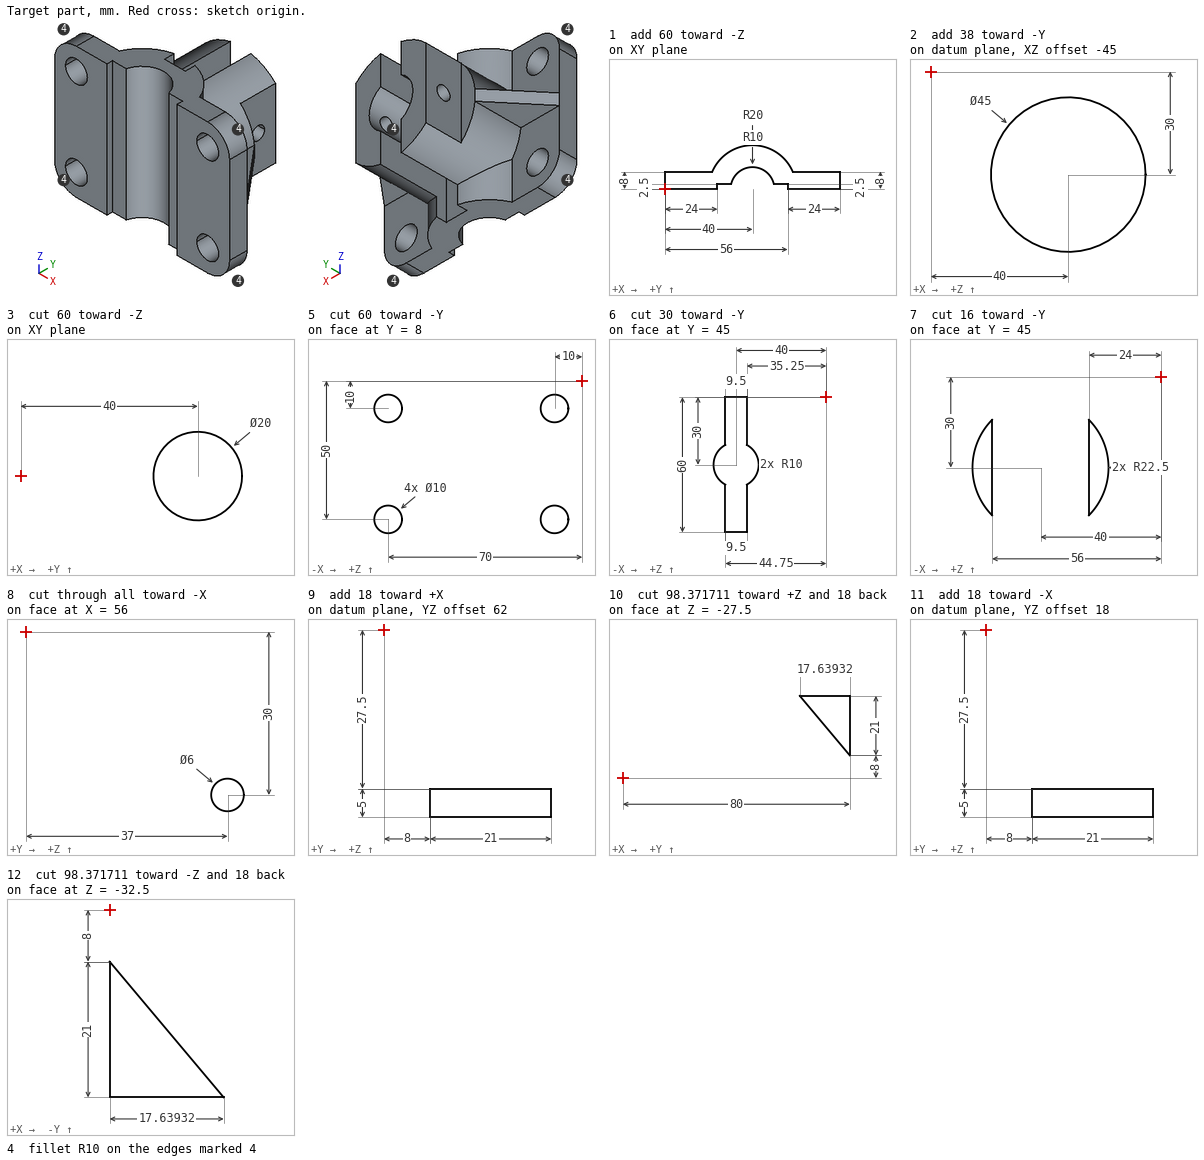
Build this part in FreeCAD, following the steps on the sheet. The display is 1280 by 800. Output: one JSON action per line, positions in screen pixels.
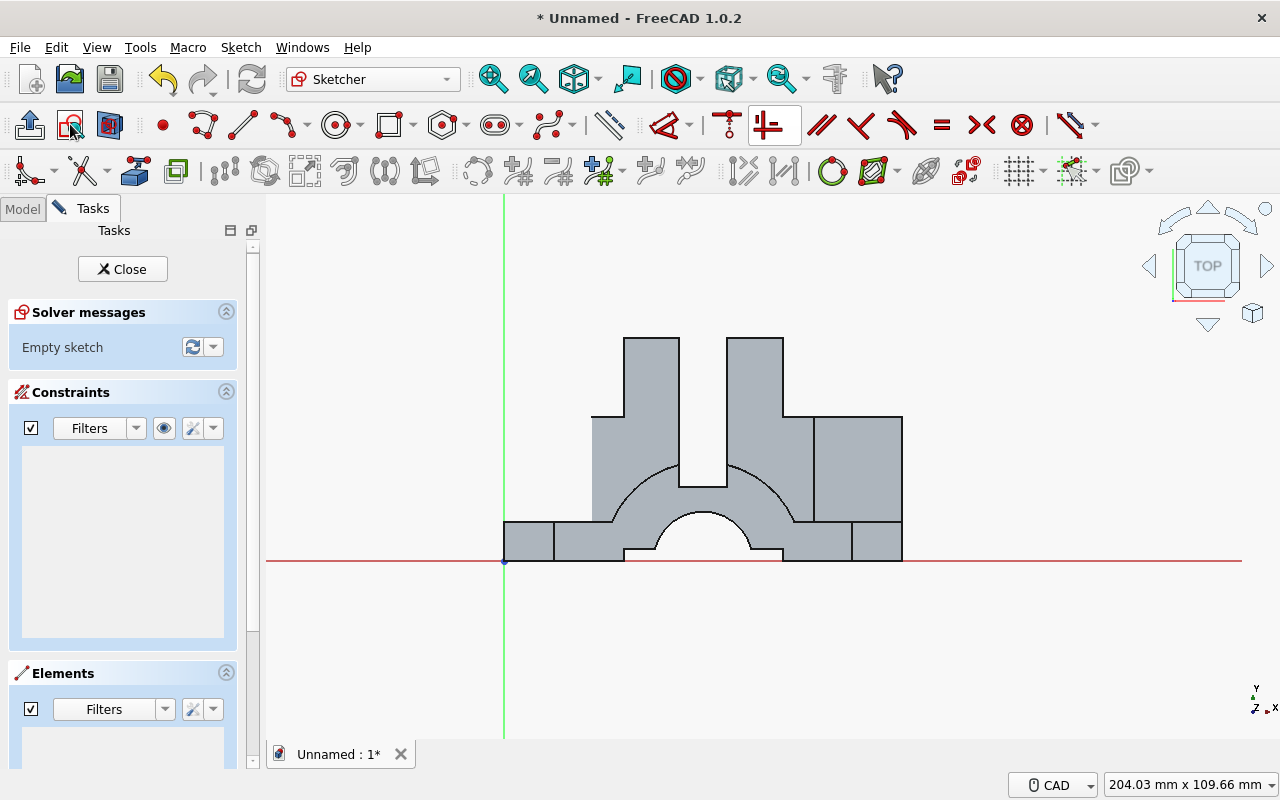
{"action": "left_click", "coordinate": [110, 126]}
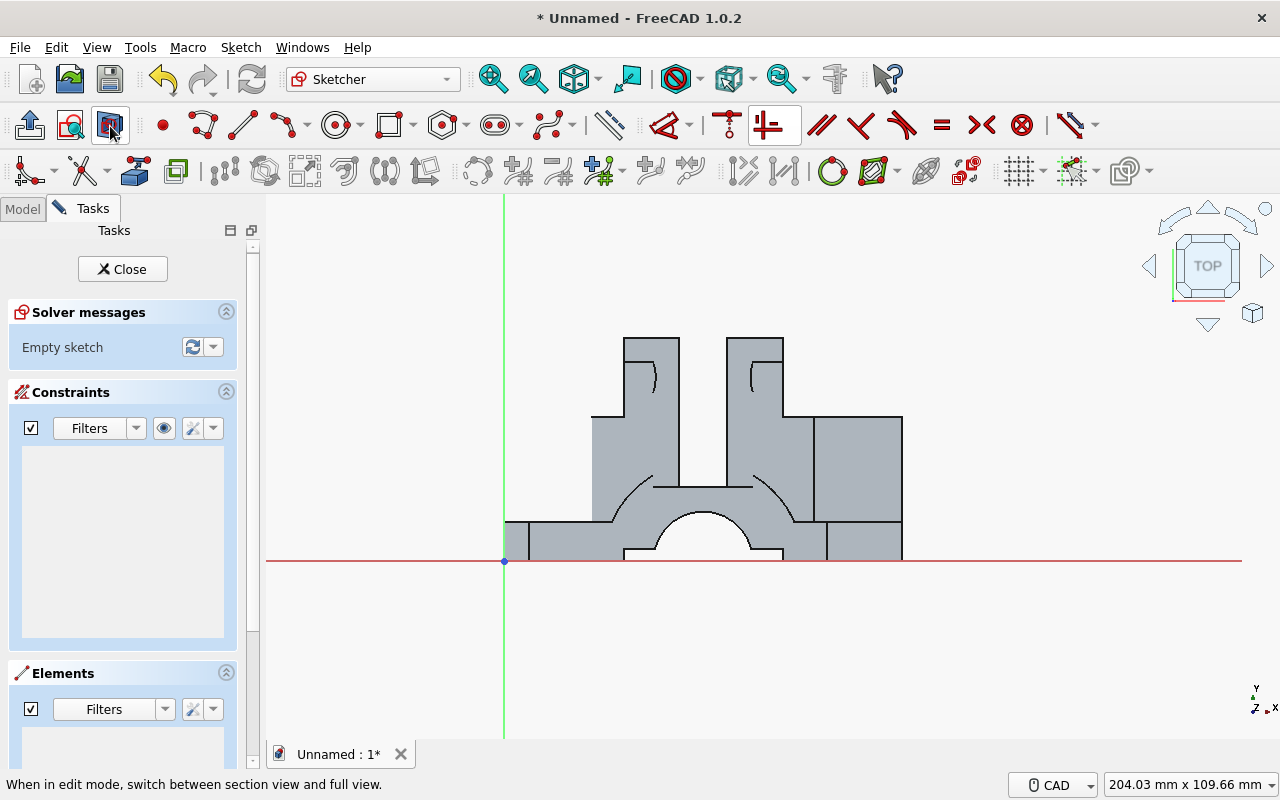
{"action": "scroll", "coordinate": [924, 471], "scroll_direction": "up", "scroll_amount": 6}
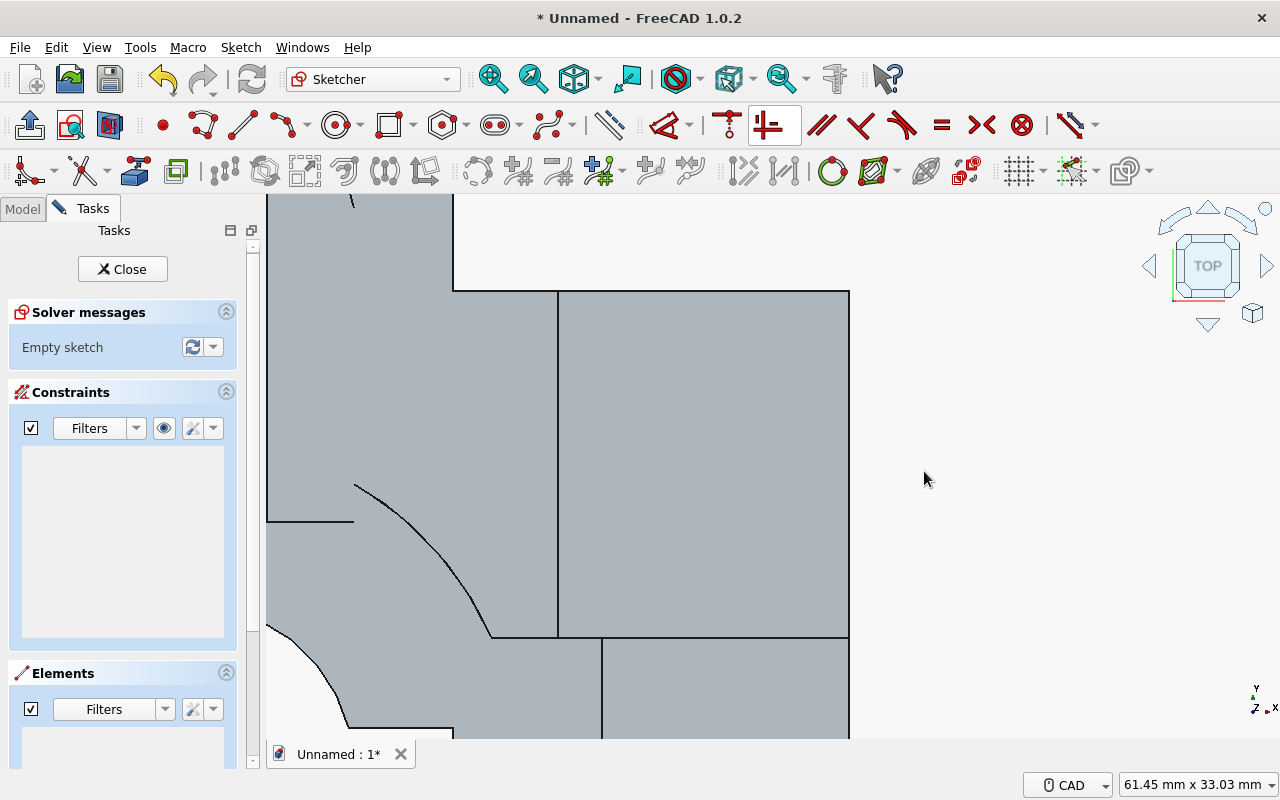
{"action": "left_click", "coordinate": [204, 126]}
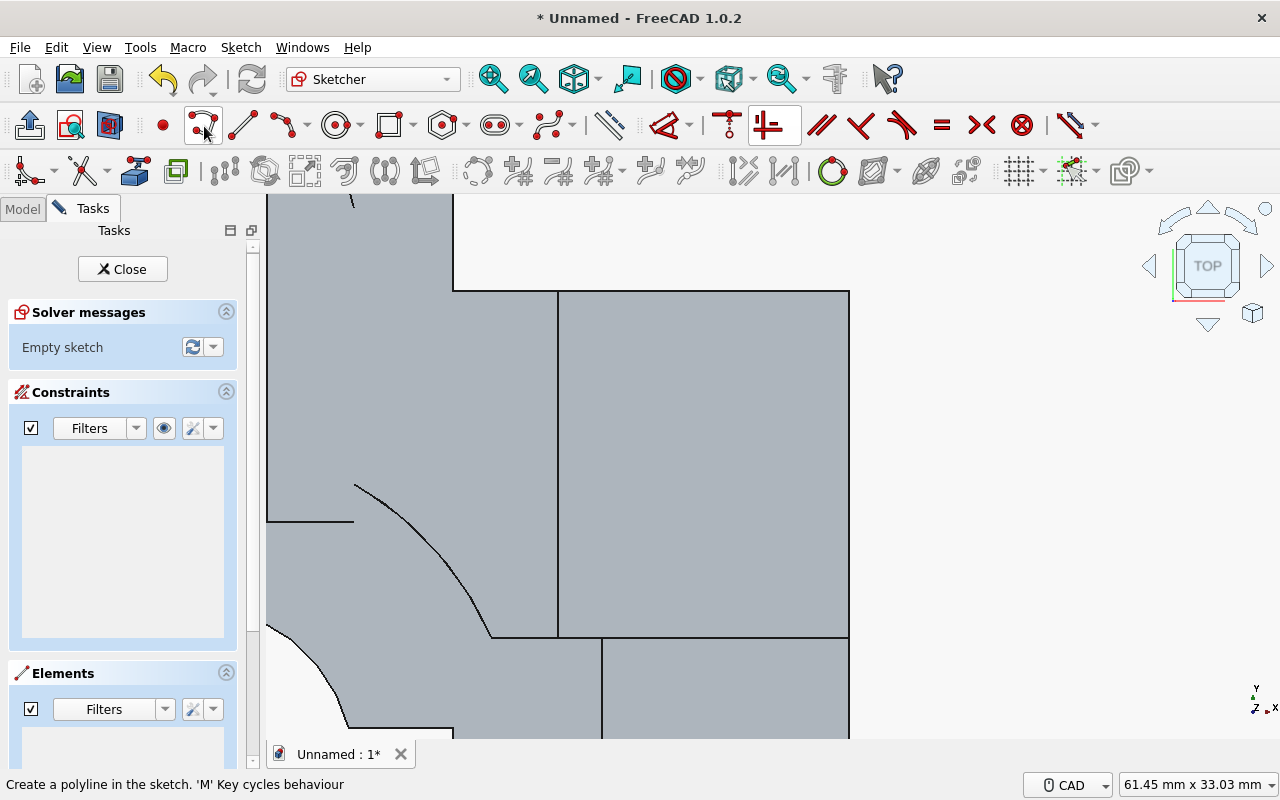
{"action": "left_click", "coordinate": [558, 291]}
{"action": "left_click", "coordinate": [849, 638]}
{"action": "left_click", "coordinate": [849, 291]}
{"action": "left_click", "coordinate": [558, 292]}
{"action": "key", "text": "Escape"}
{"action": "key", "text": "Escape"}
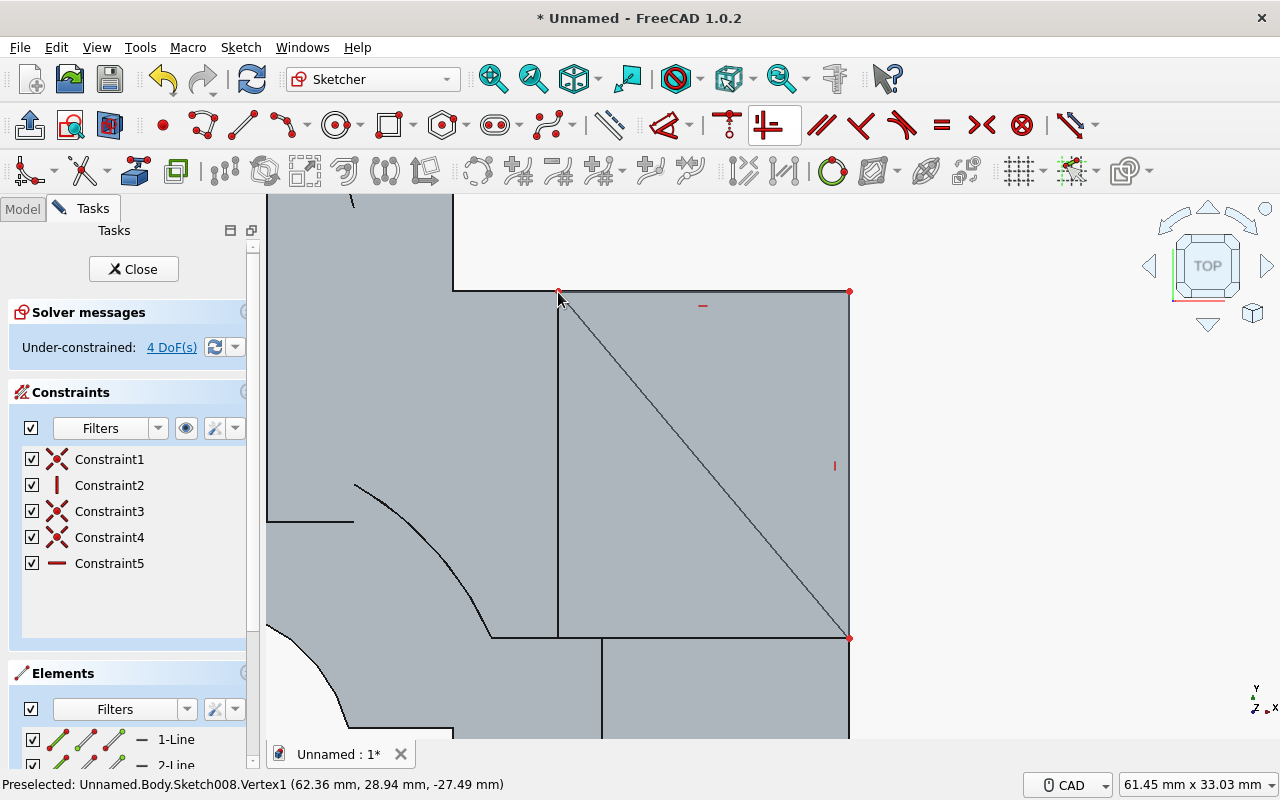
{"action": "left_click", "coordinate": [664, 126]}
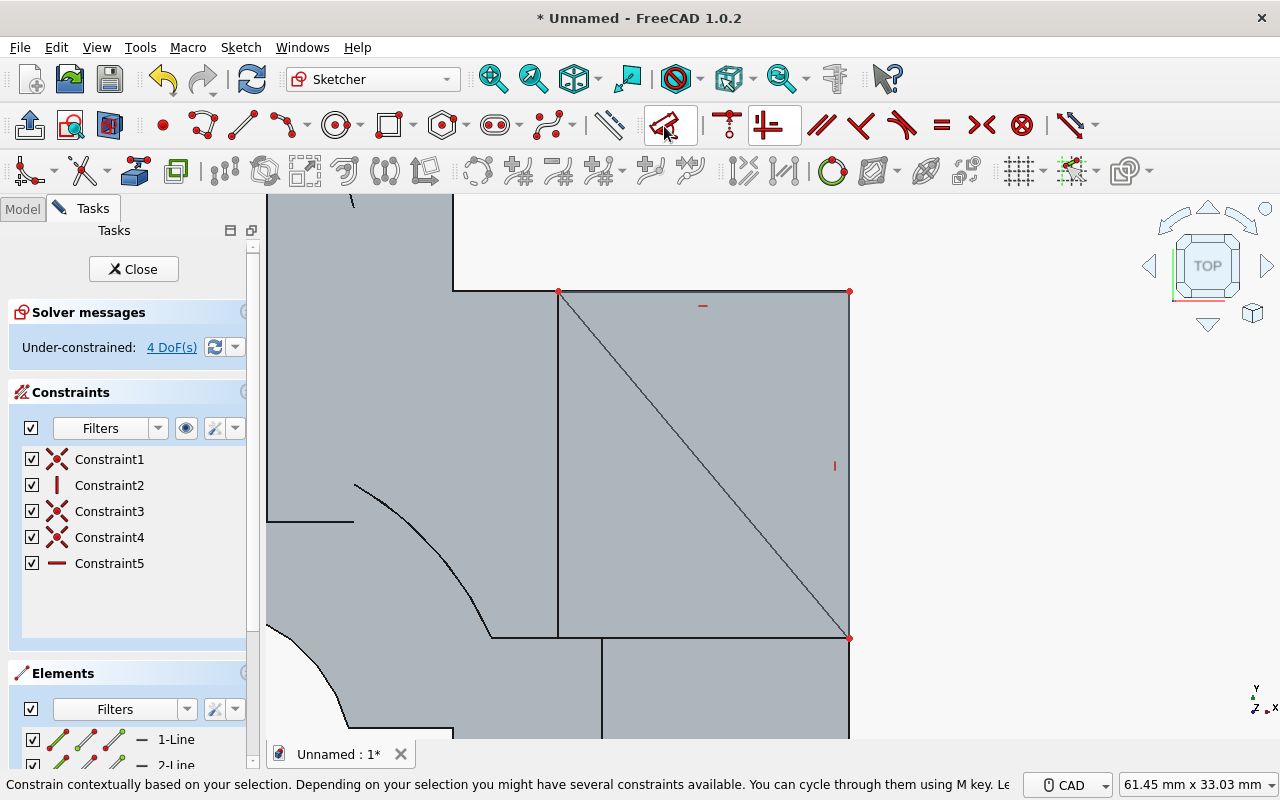
{"action": "left_click", "coordinate": [849, 535]}
{"action": "left_click", "coordinate": [883, 465]}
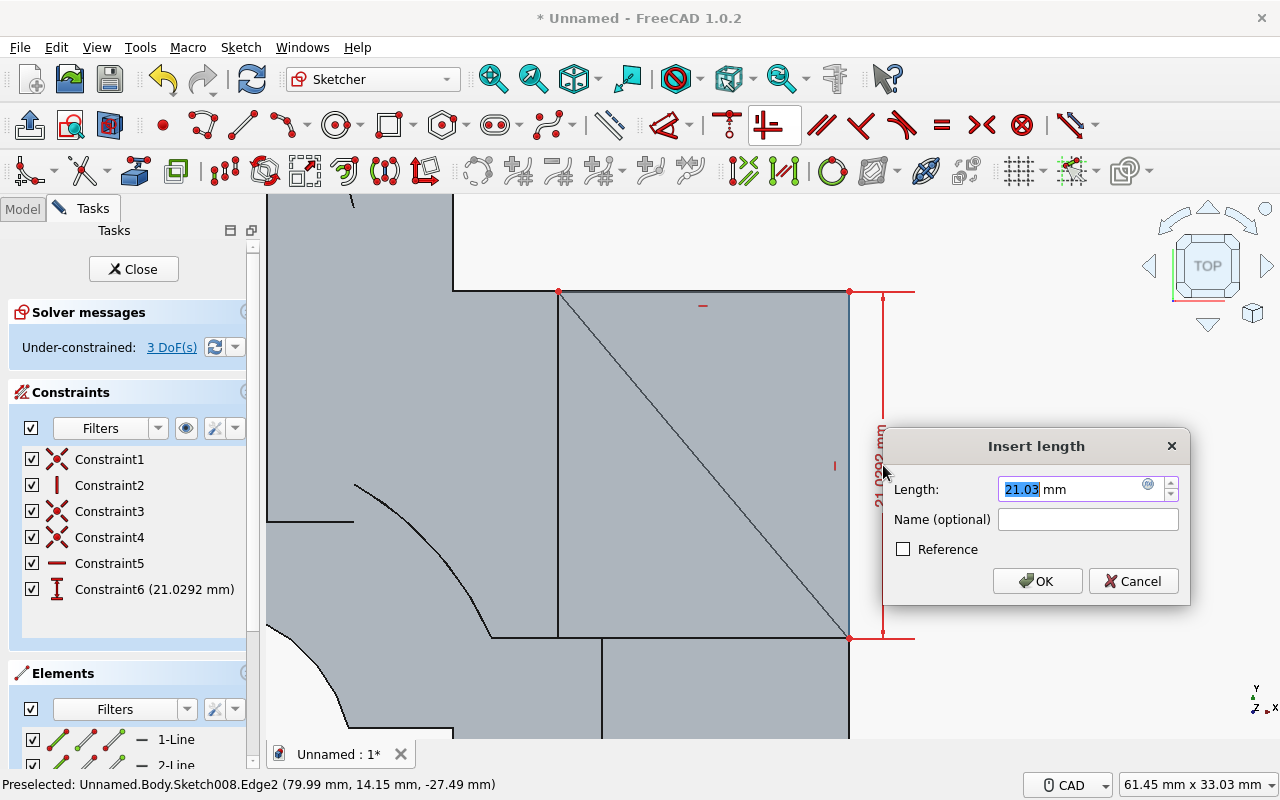
{"action": "type", "text": "21"}
{"action": "key", "text": "Return"}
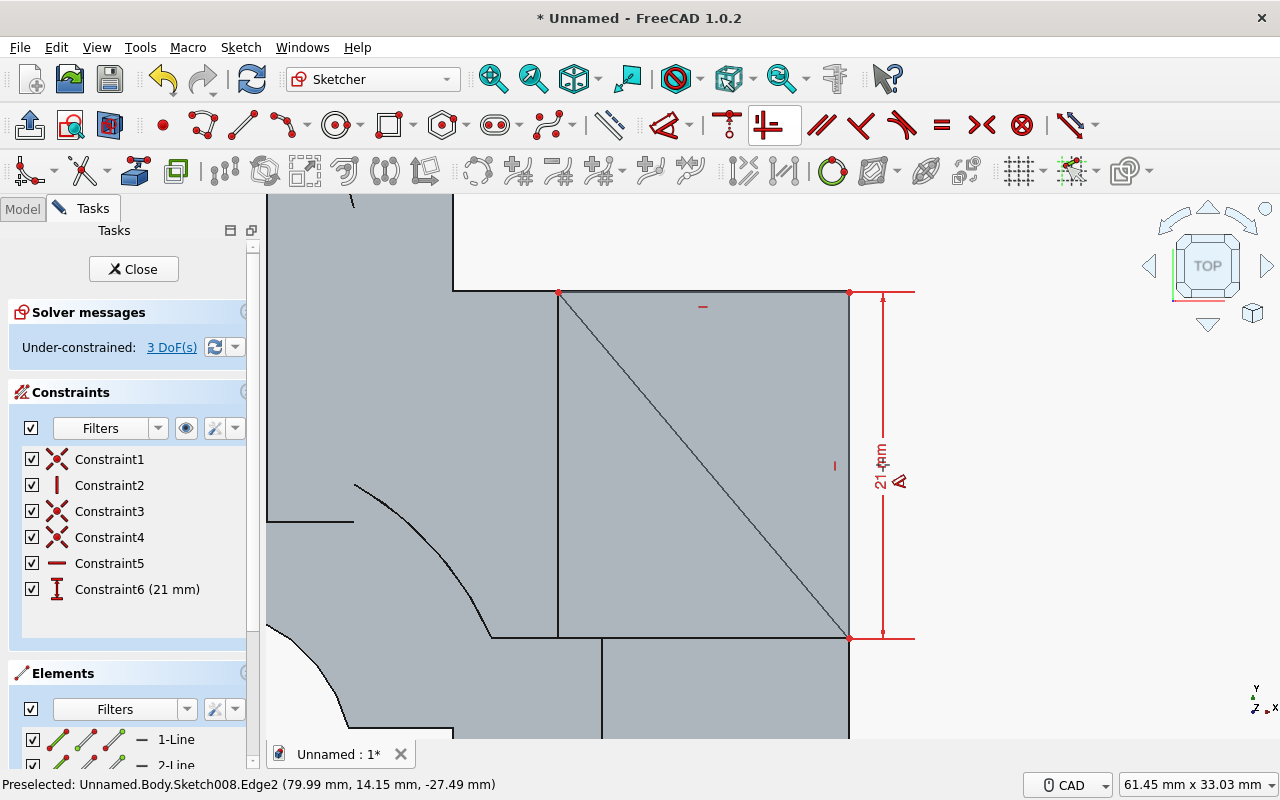
{"action": "left_click", "coordinate": [849, 639]}
{"action": "left_click", "coordinate": [883, 675]}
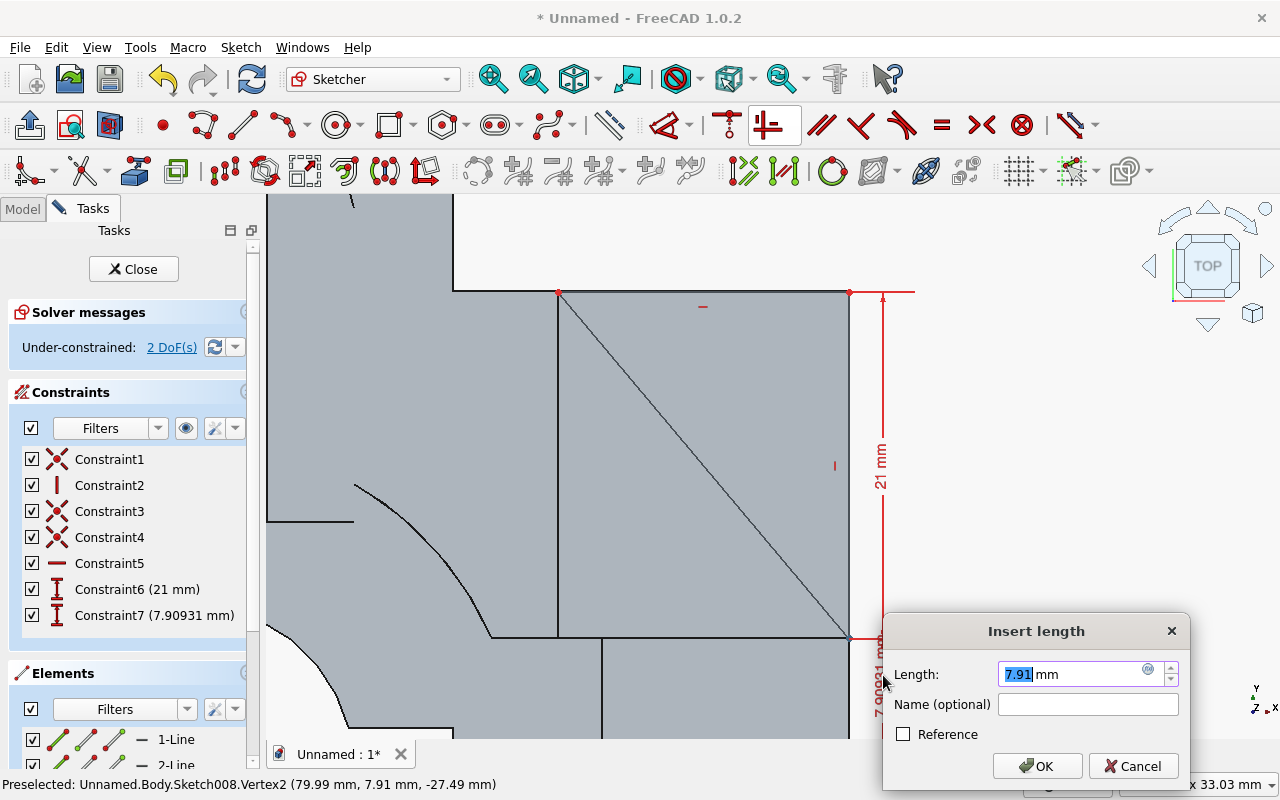
{"action": "type", "text": "8"}
{"action": "key", "text": "Return"}